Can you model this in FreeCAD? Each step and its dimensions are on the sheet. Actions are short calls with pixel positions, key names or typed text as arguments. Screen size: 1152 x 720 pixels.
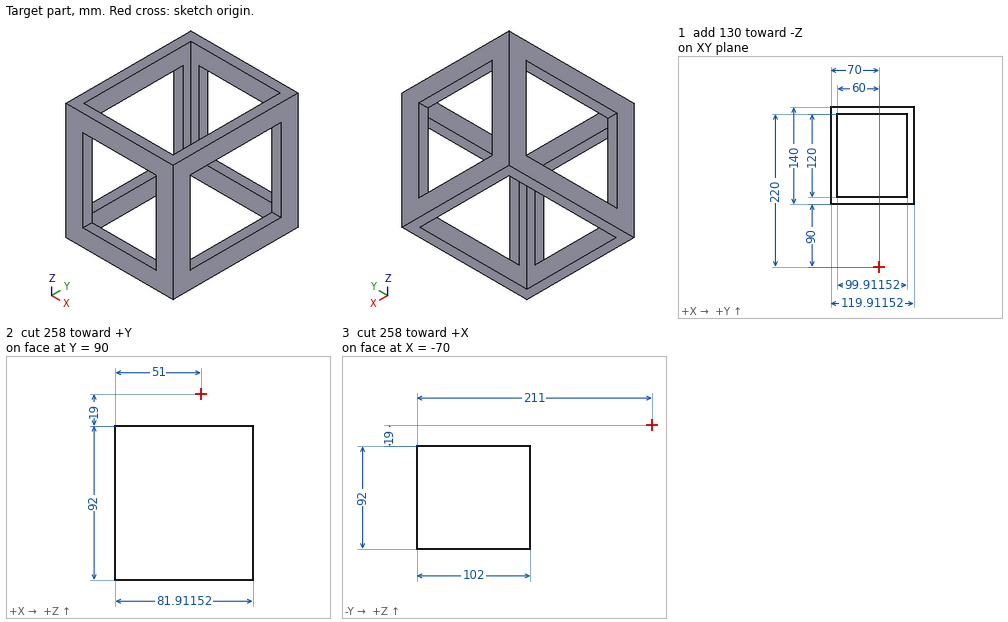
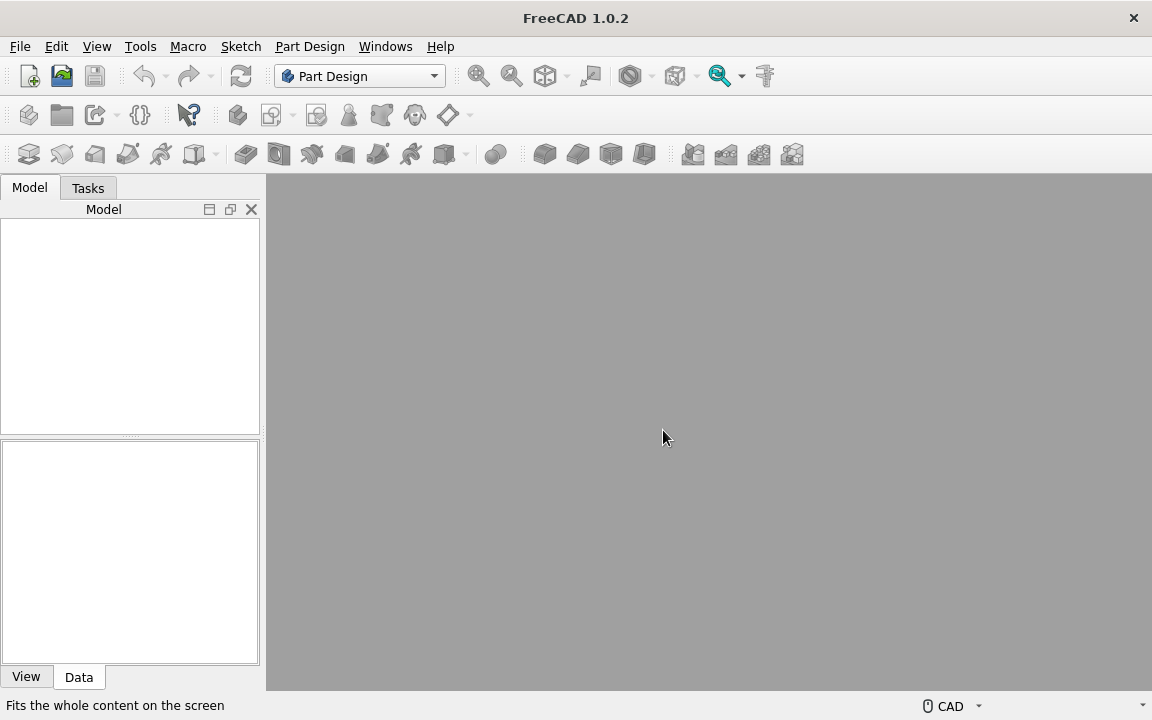
click(29, 76)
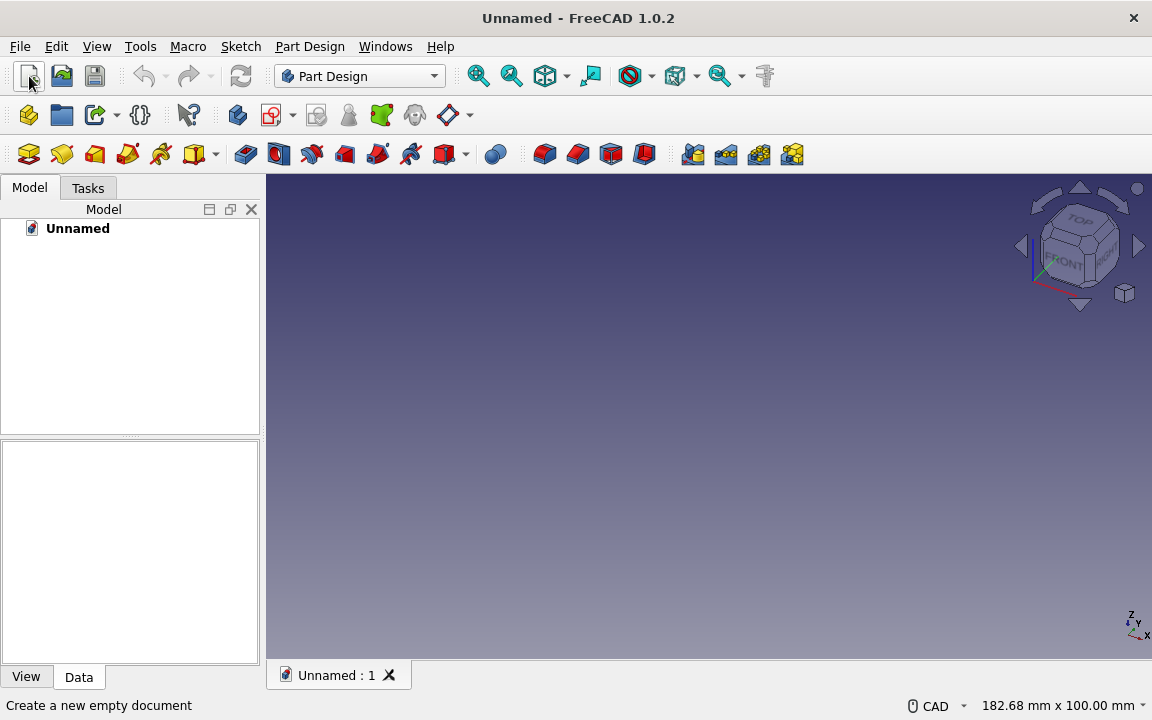
click(270, 116)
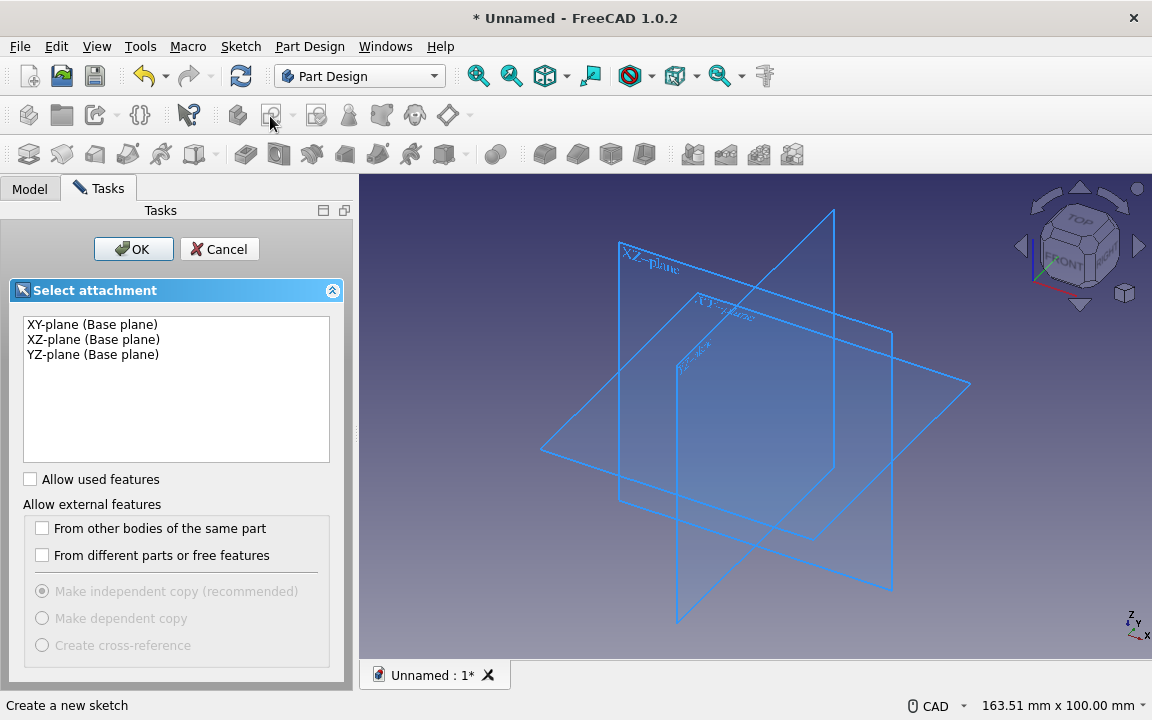
click(84, 324)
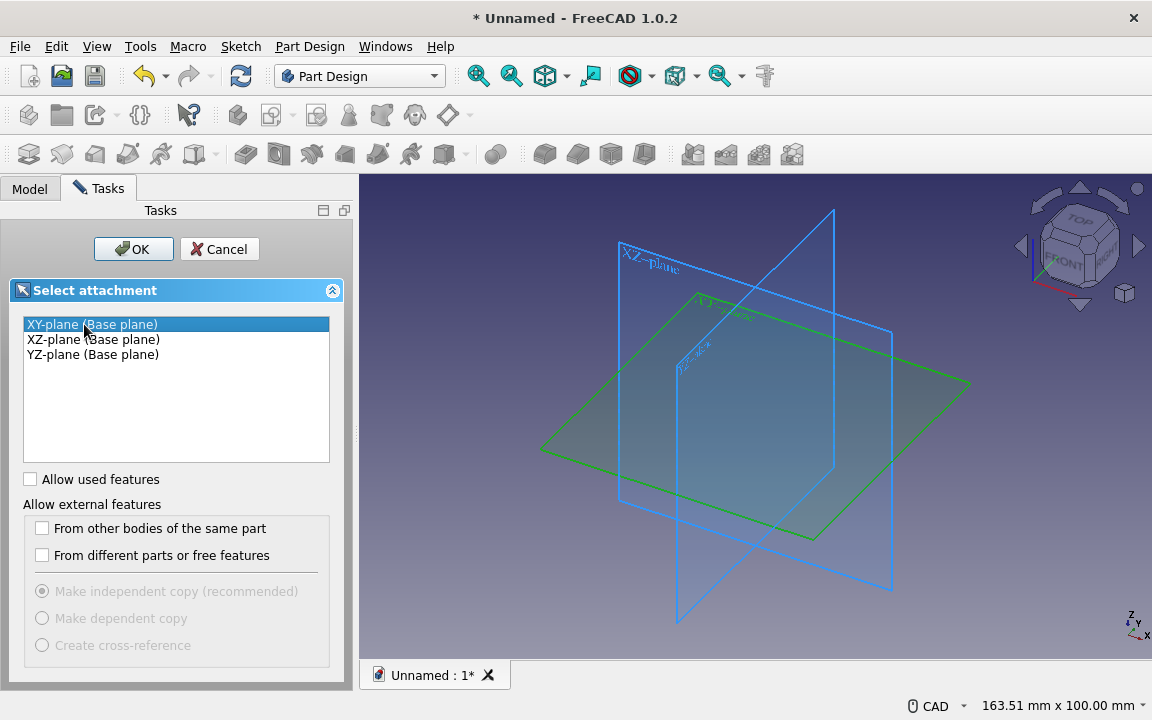
click(134, 249)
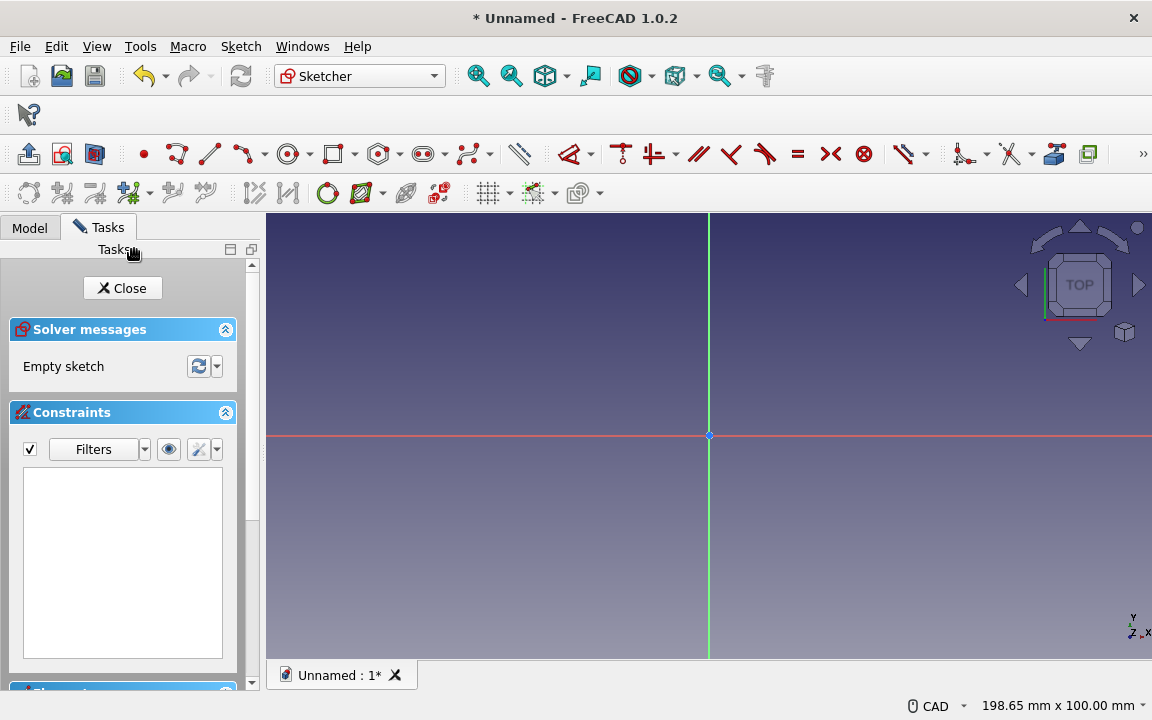
scroll(633, 604, down, 7)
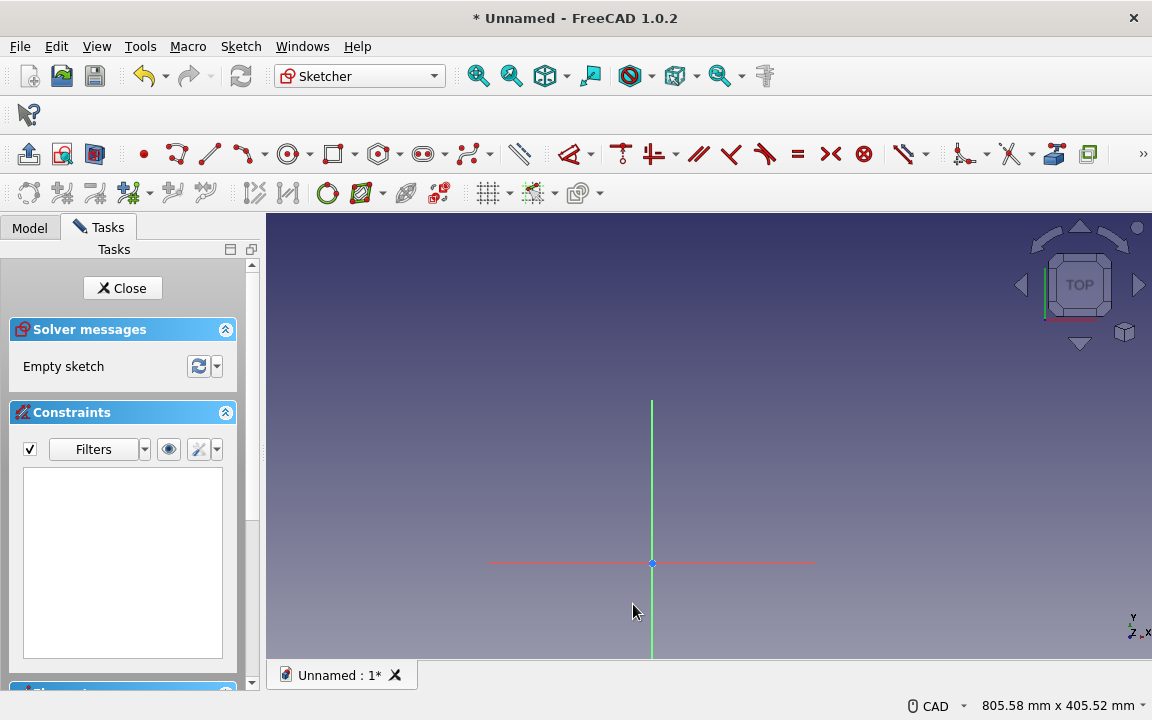
key(g)
key(r)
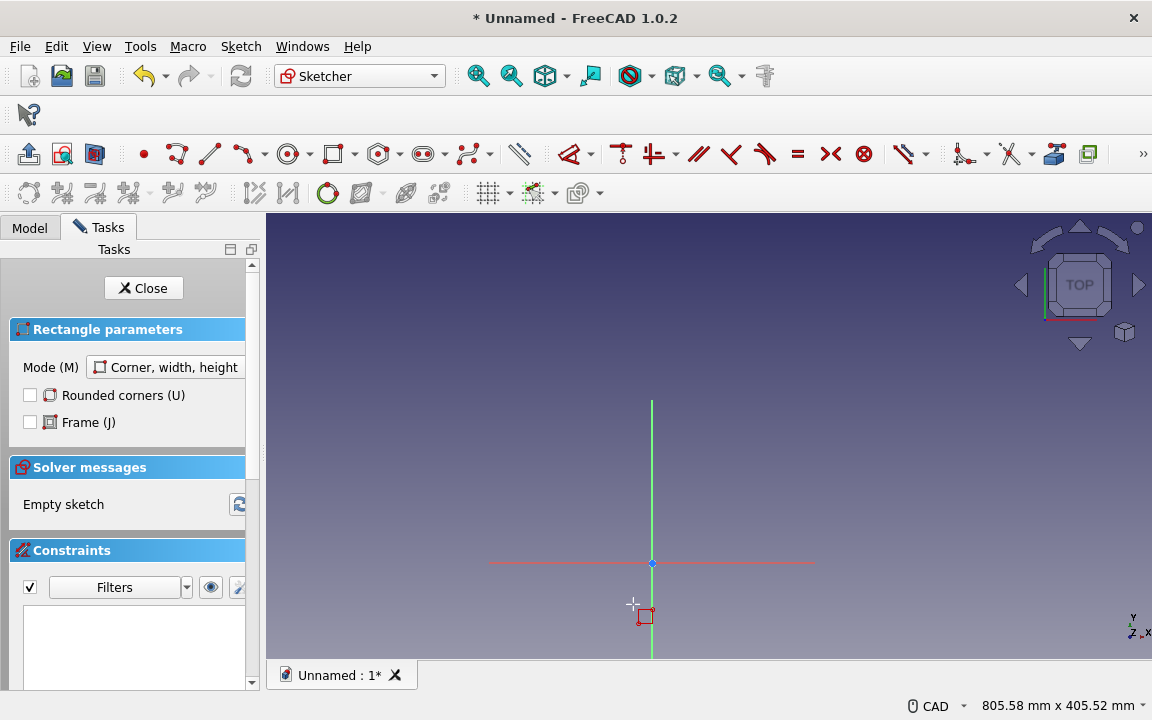
click(575, 310)
click(707, 464)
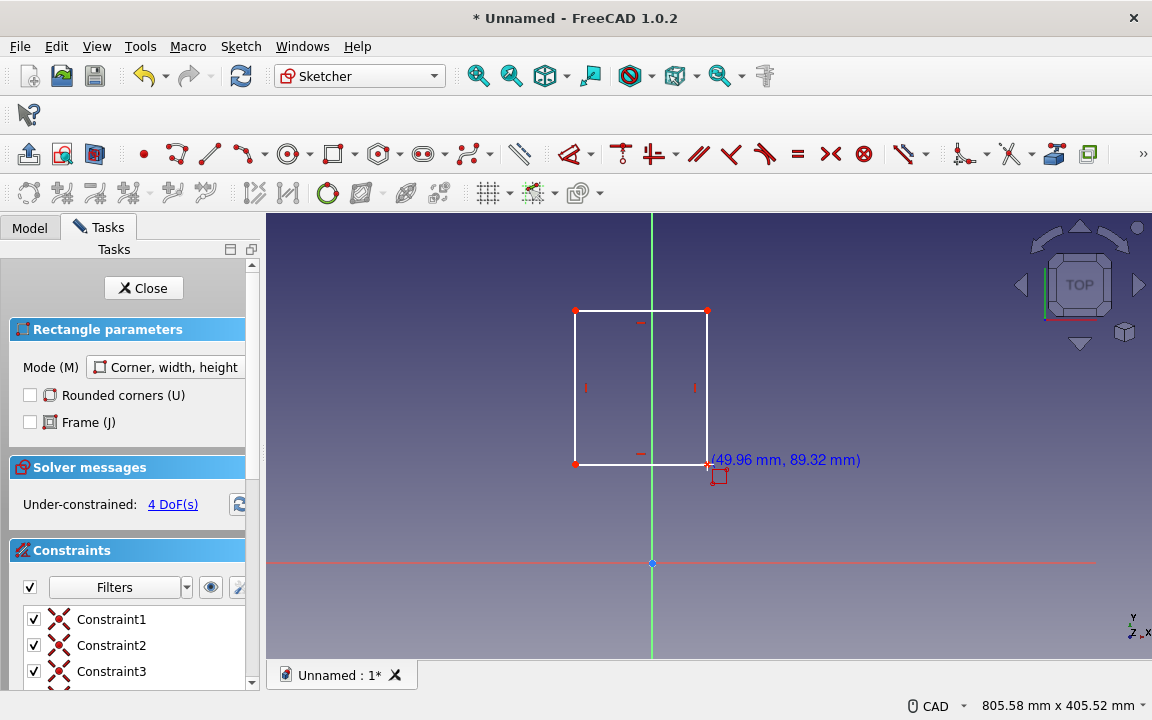
scroll(586, 321, up, 2)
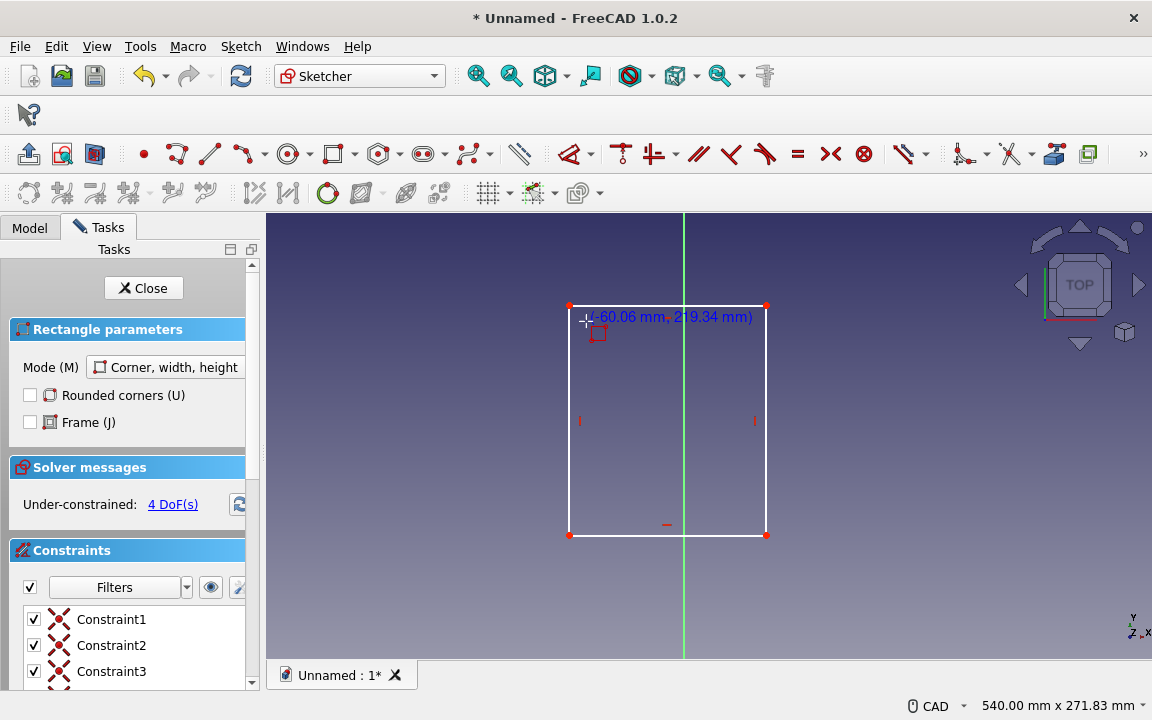
click(586, 321)
click(750, 518)
key(Escape)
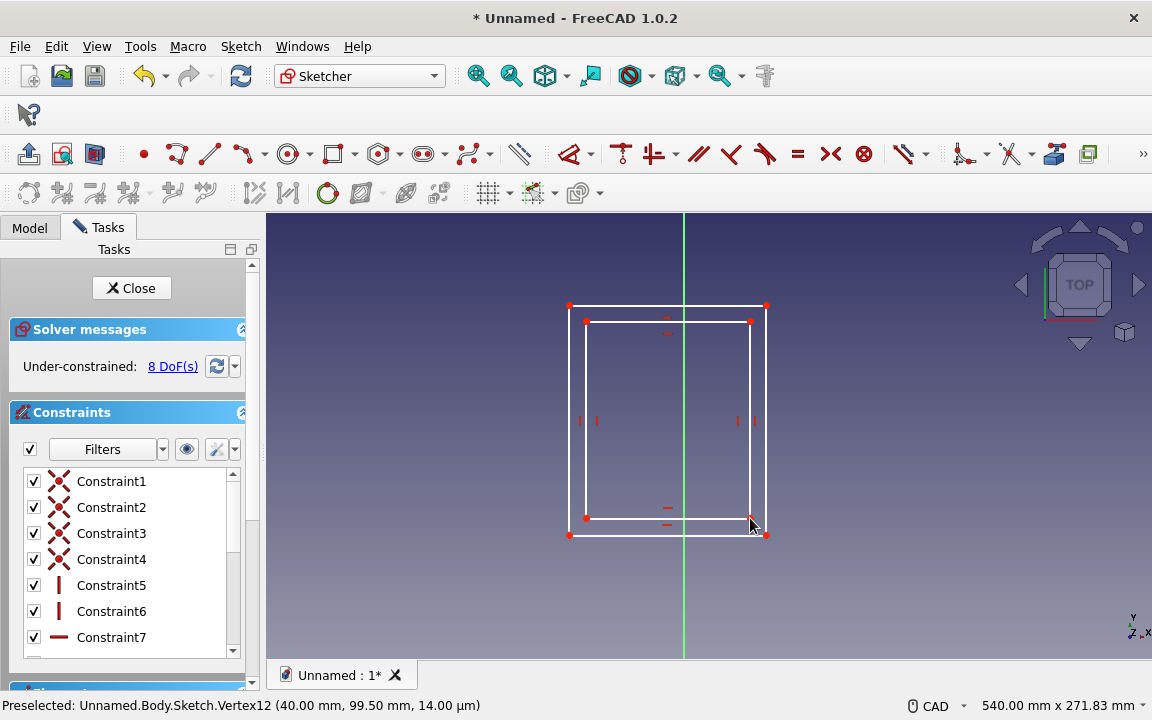
click(569, 375)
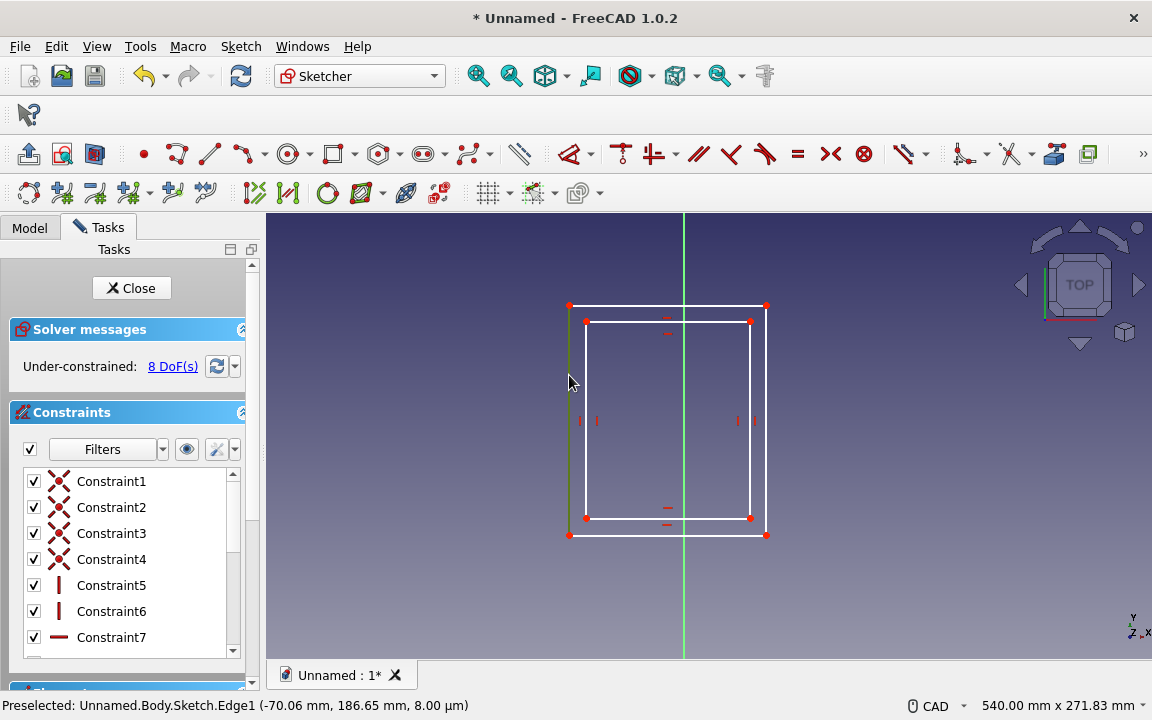
key(i)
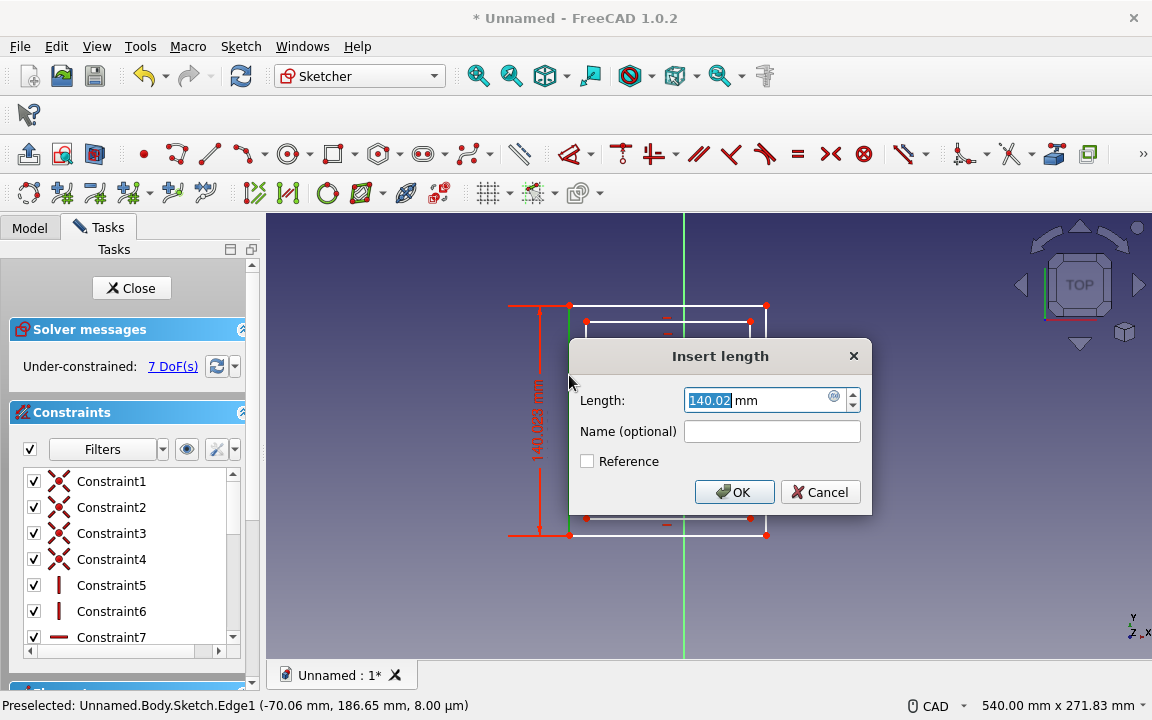
text(140)
key(Return)